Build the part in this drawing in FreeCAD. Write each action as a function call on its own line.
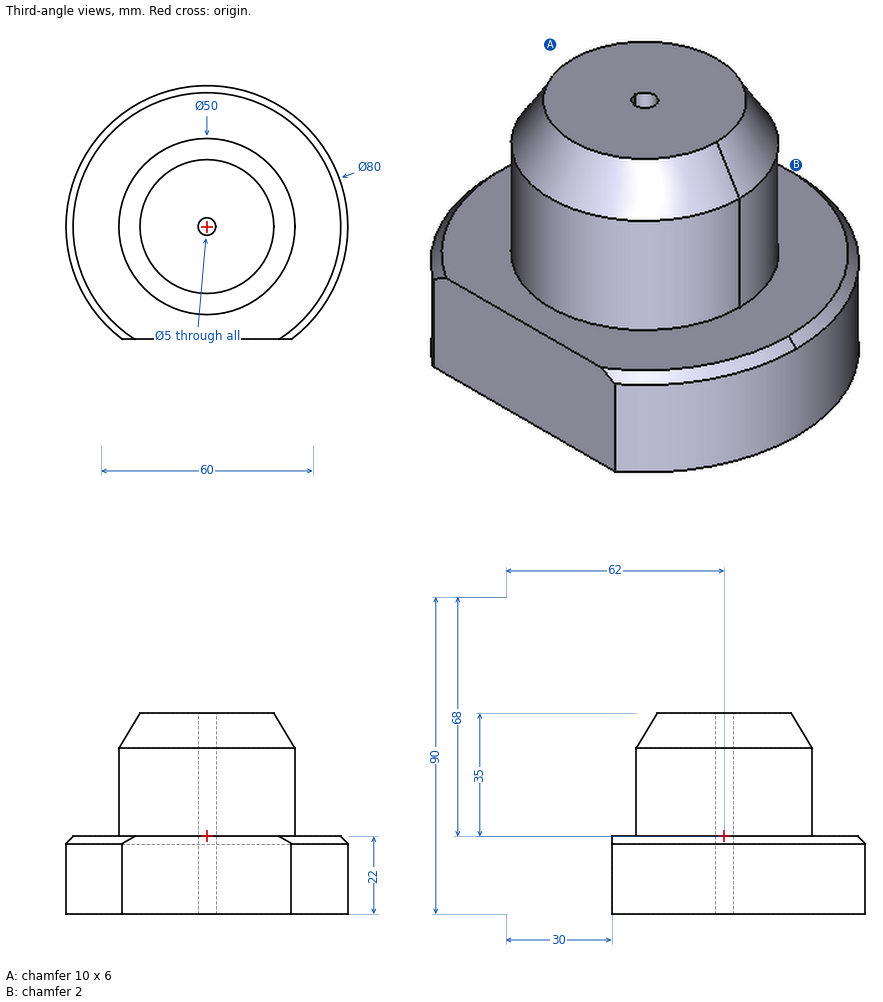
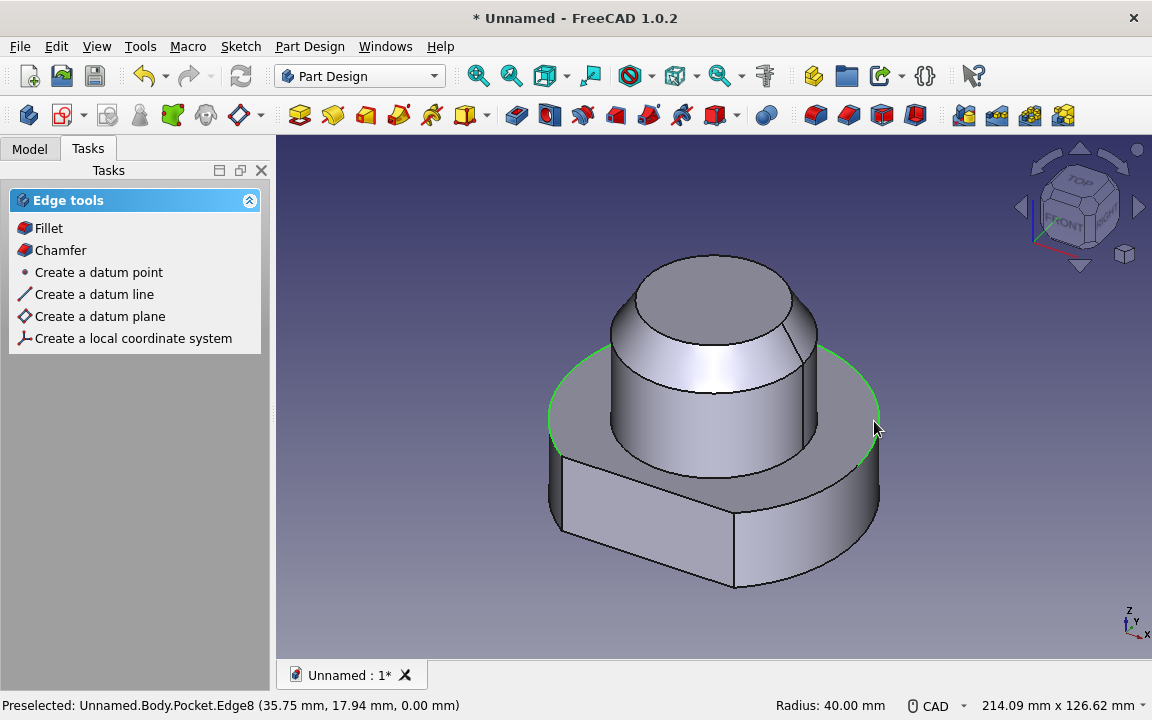
click(849, 116)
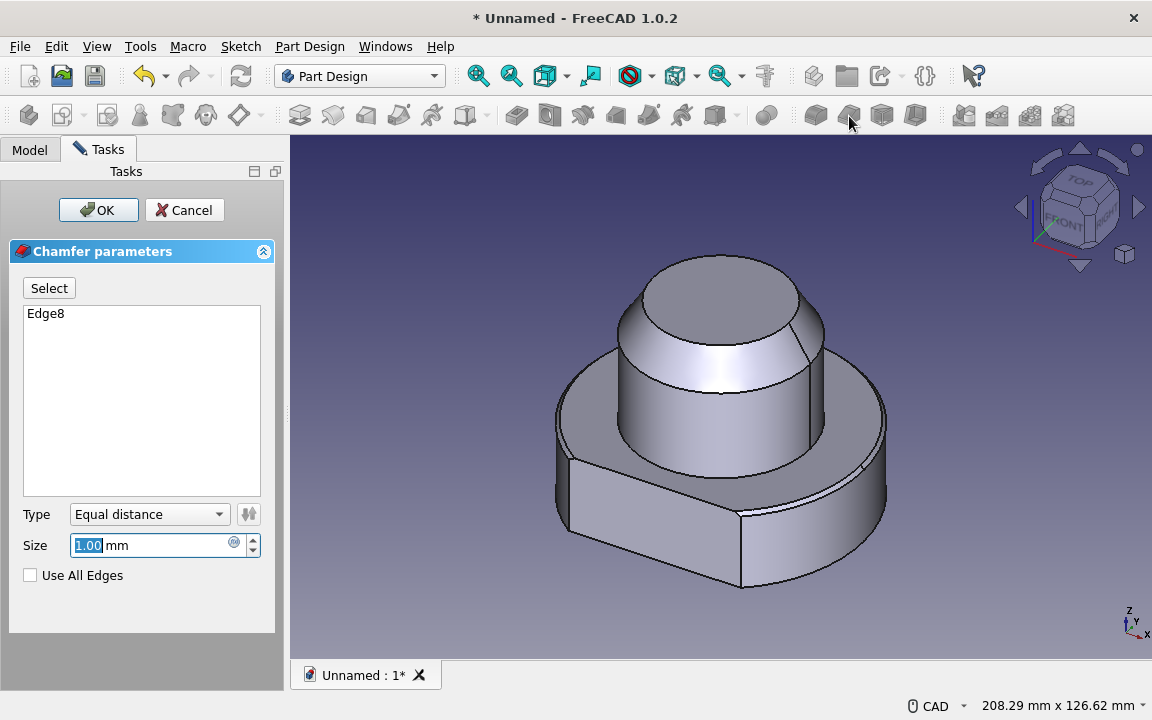
text(2)
key(Tab)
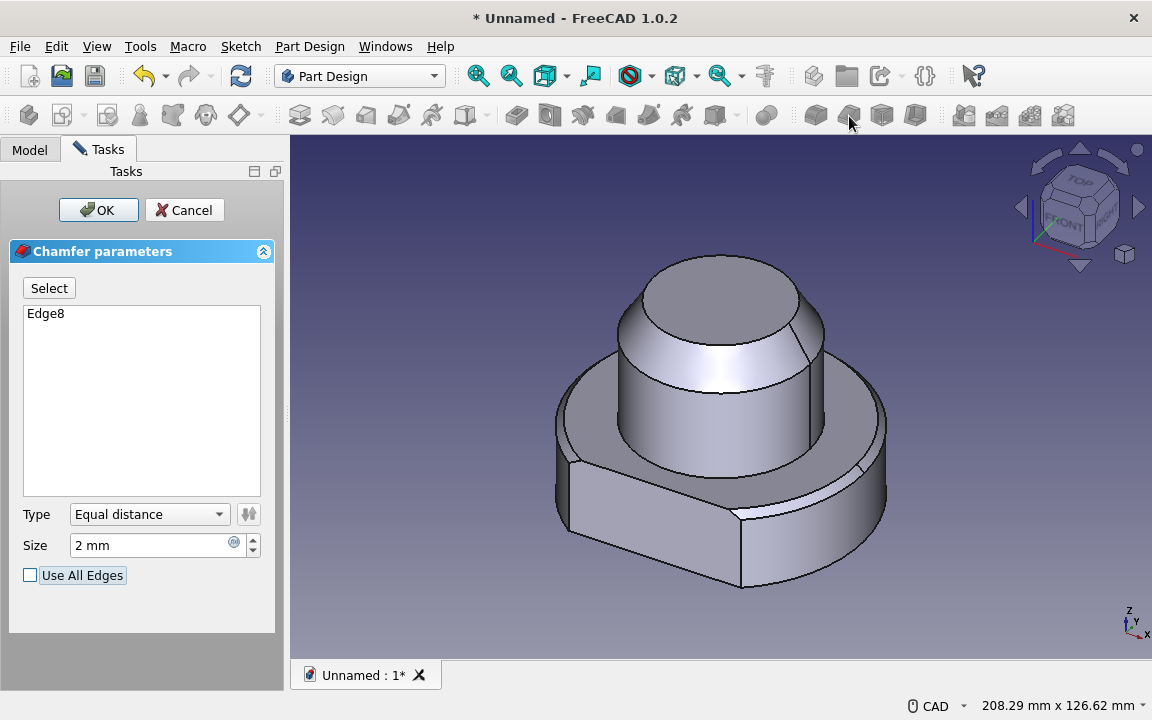
click(99, 210)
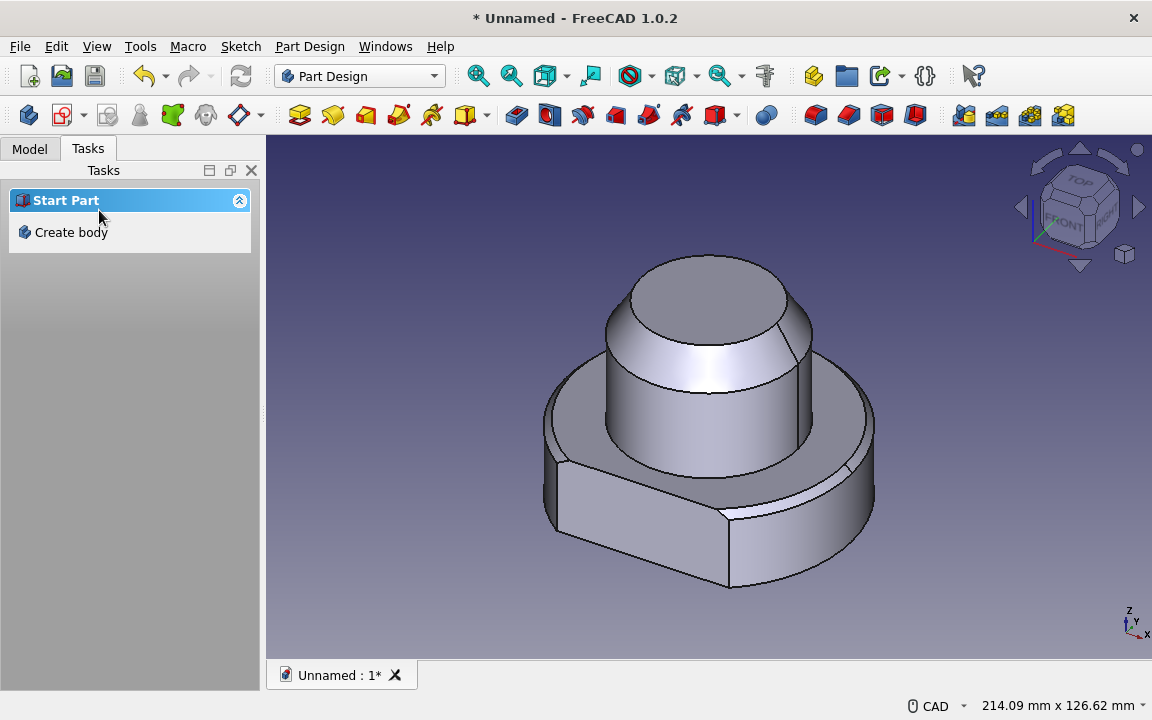
key(5)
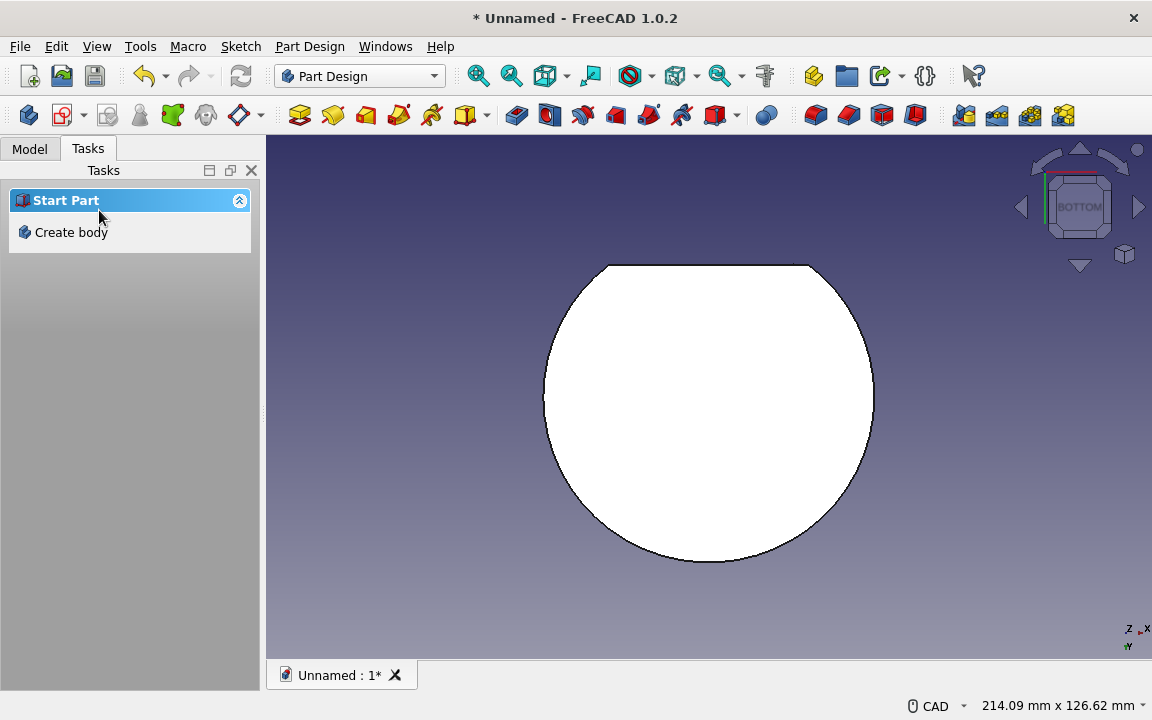
click(709, 413)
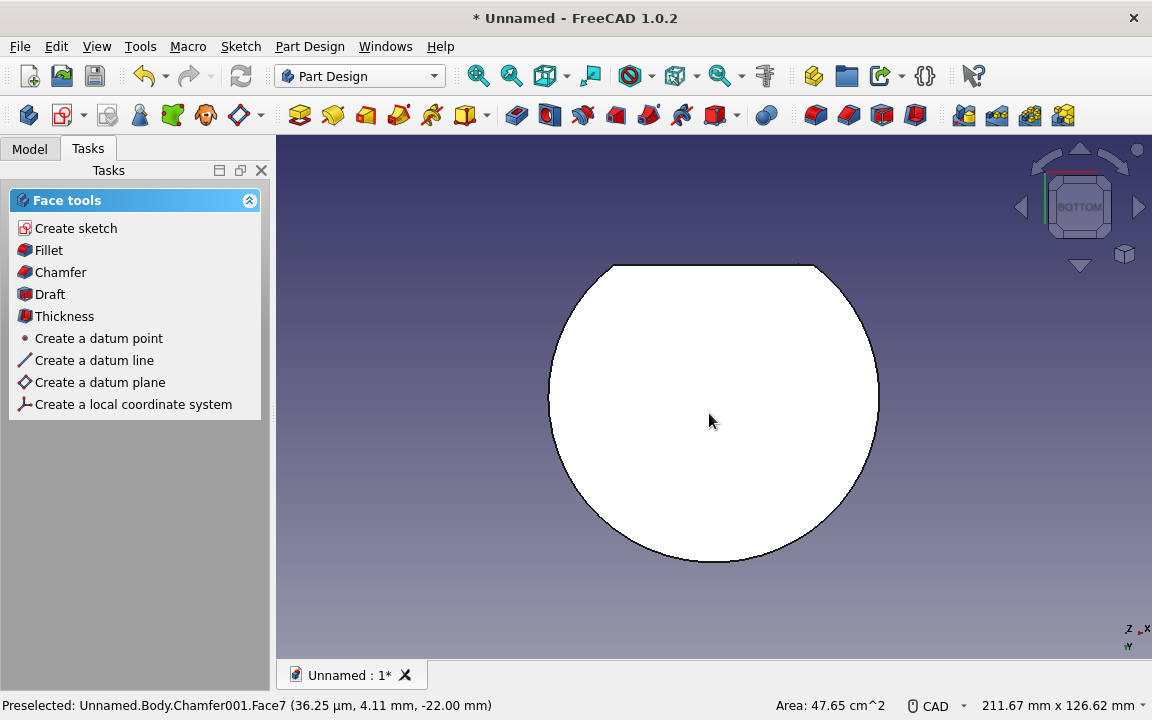
click(62, 116)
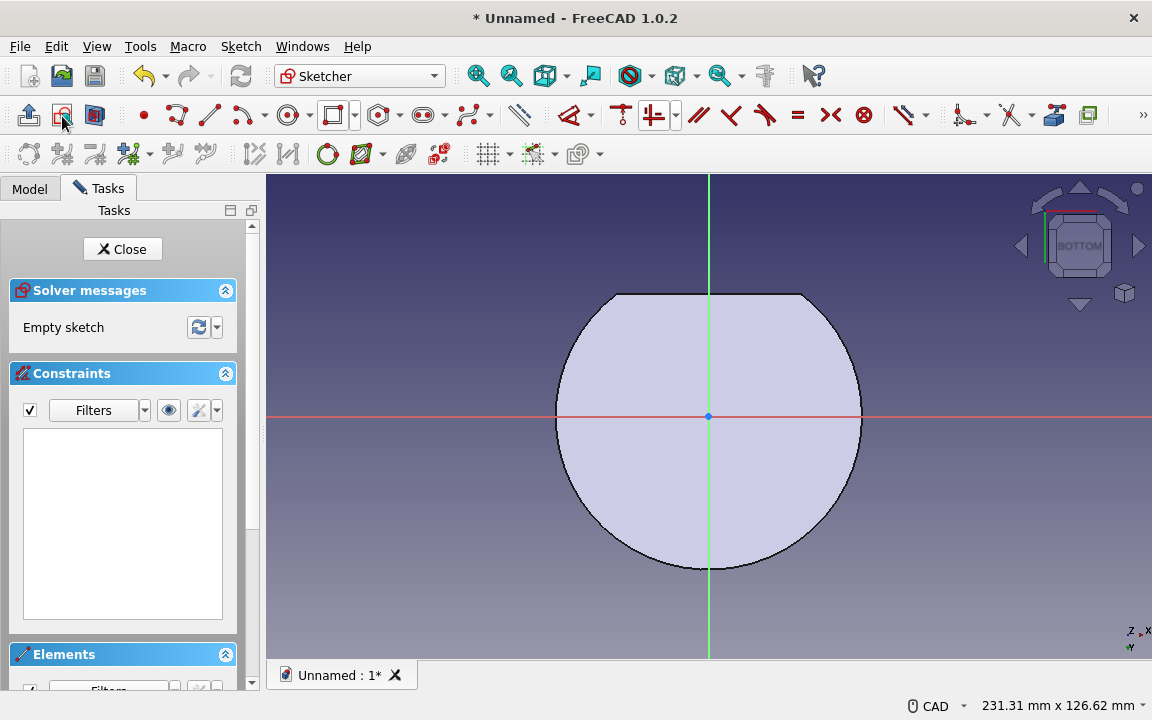
scroll(713, 417, up, 14)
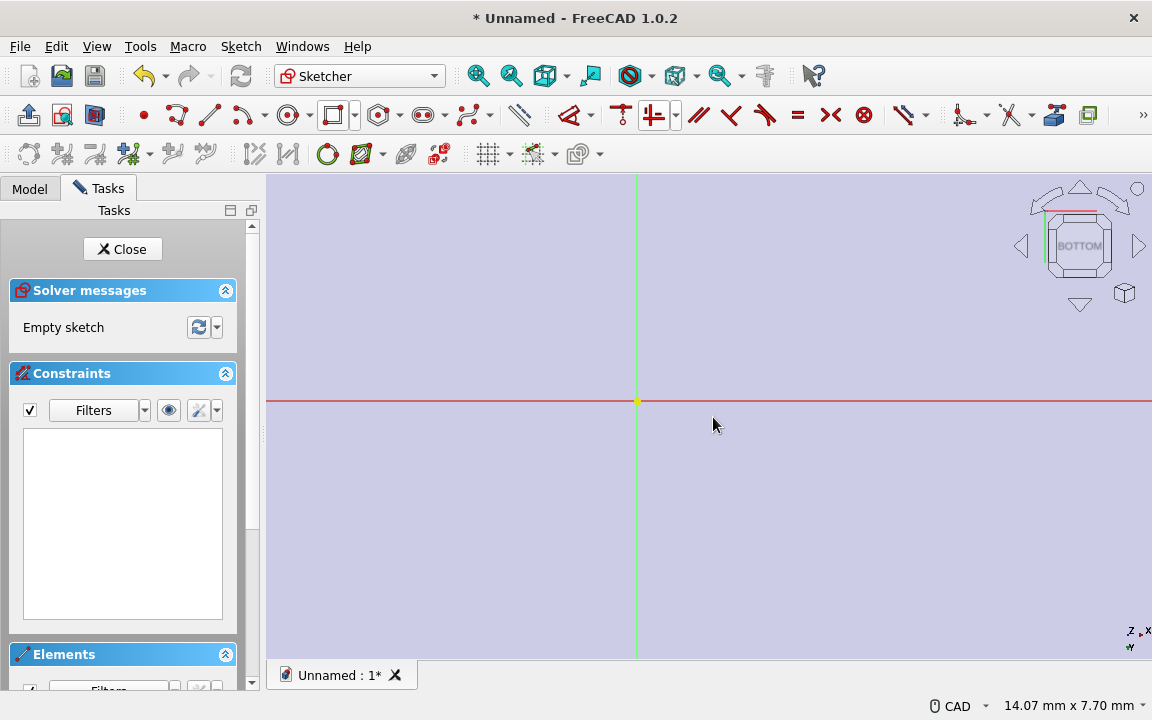
click(288, 116)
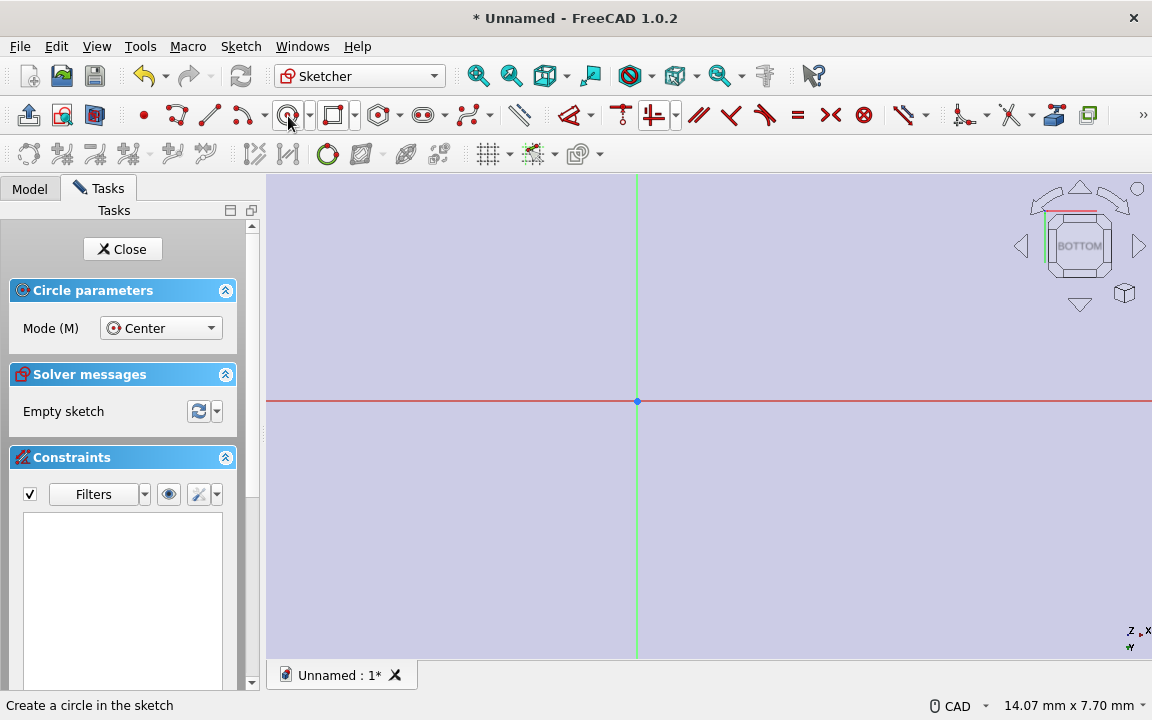
click(637, 401)
click(748, 290)
key(Escape)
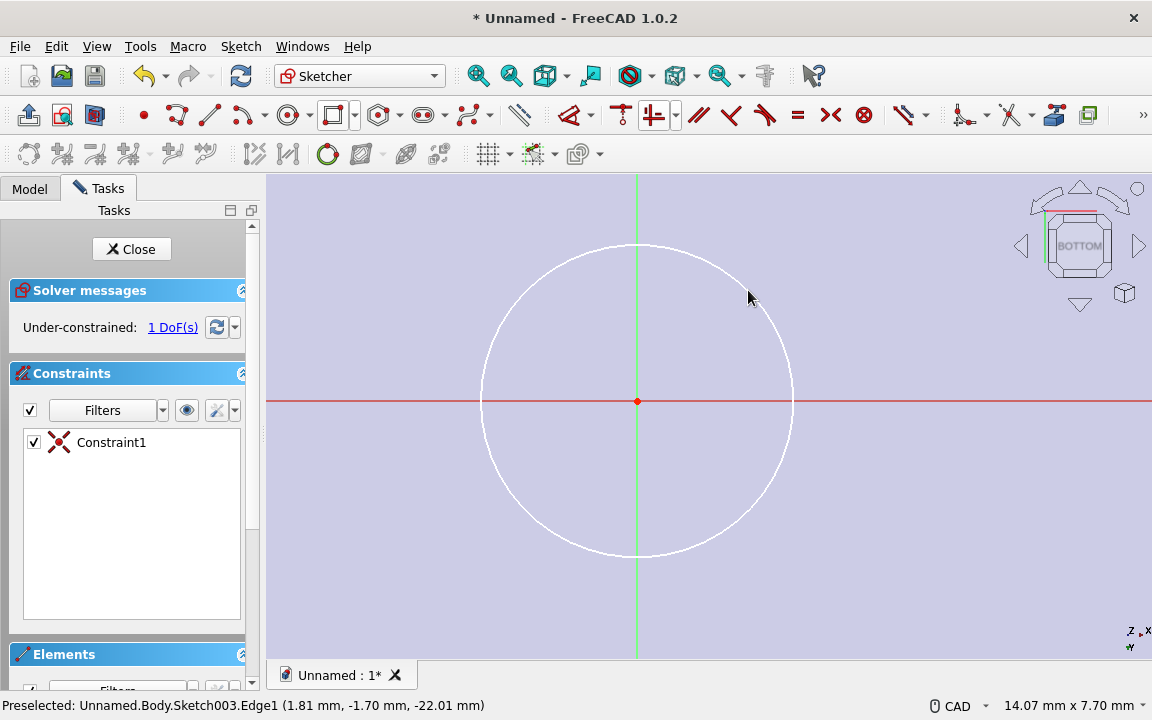
key(d)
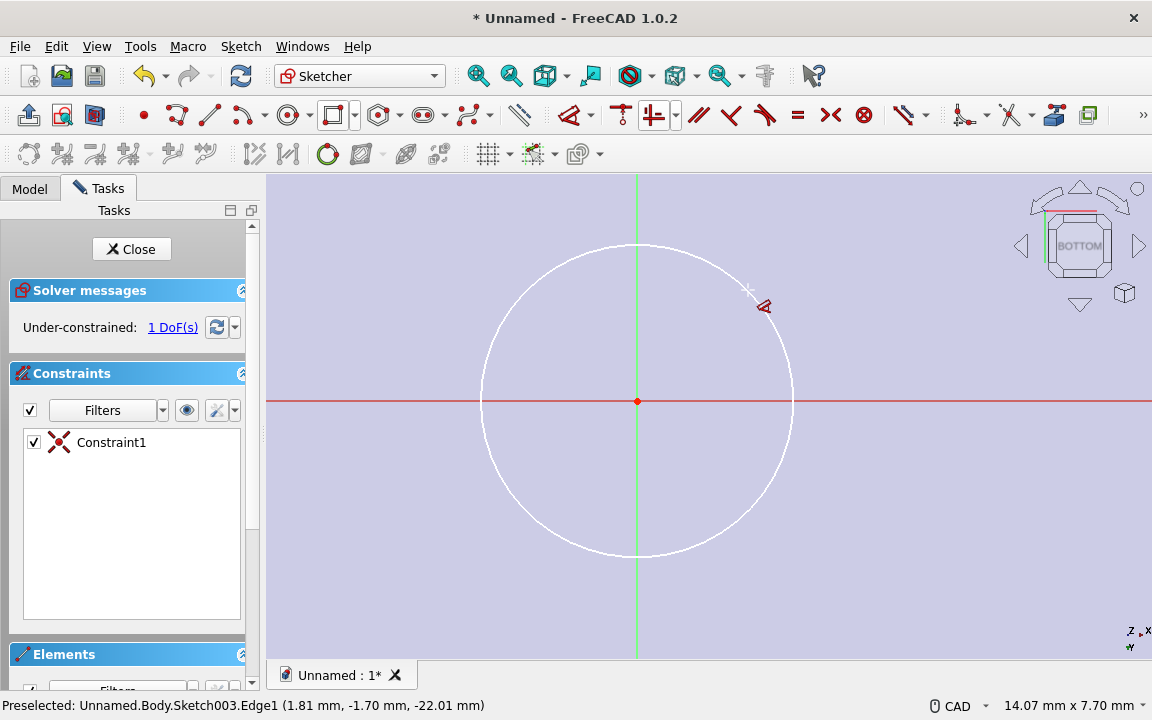
click(747, 290)
click(769, 267)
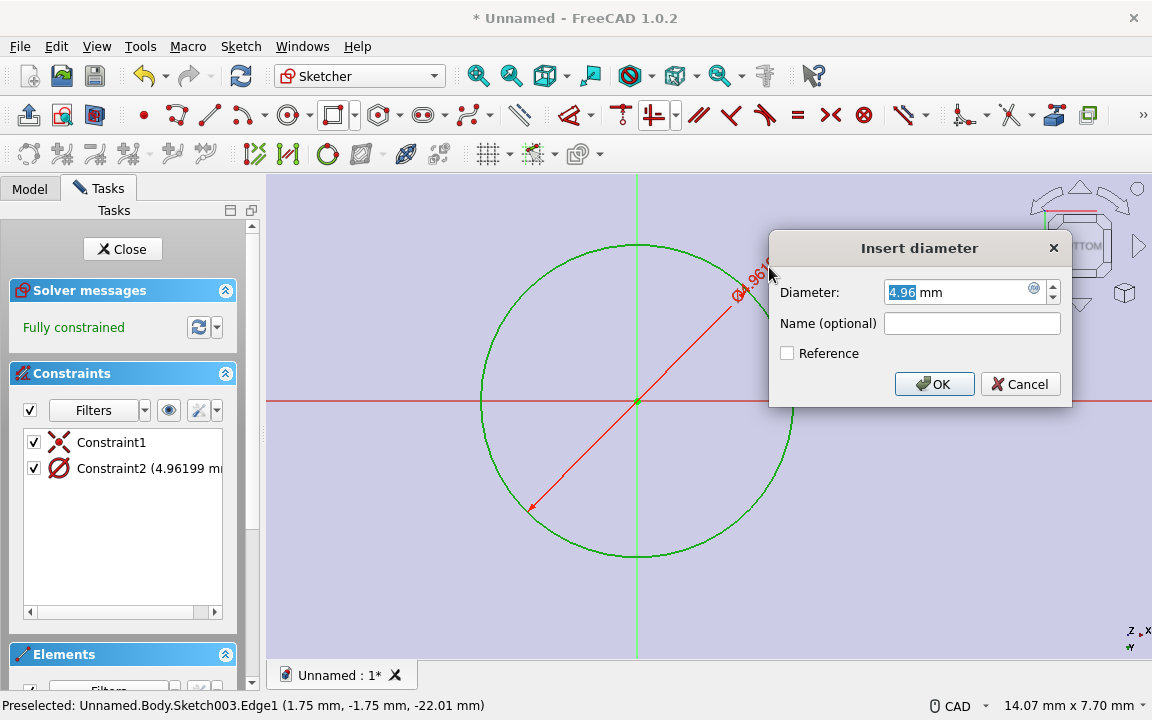
text(5)
key(Return)
key(Escape)